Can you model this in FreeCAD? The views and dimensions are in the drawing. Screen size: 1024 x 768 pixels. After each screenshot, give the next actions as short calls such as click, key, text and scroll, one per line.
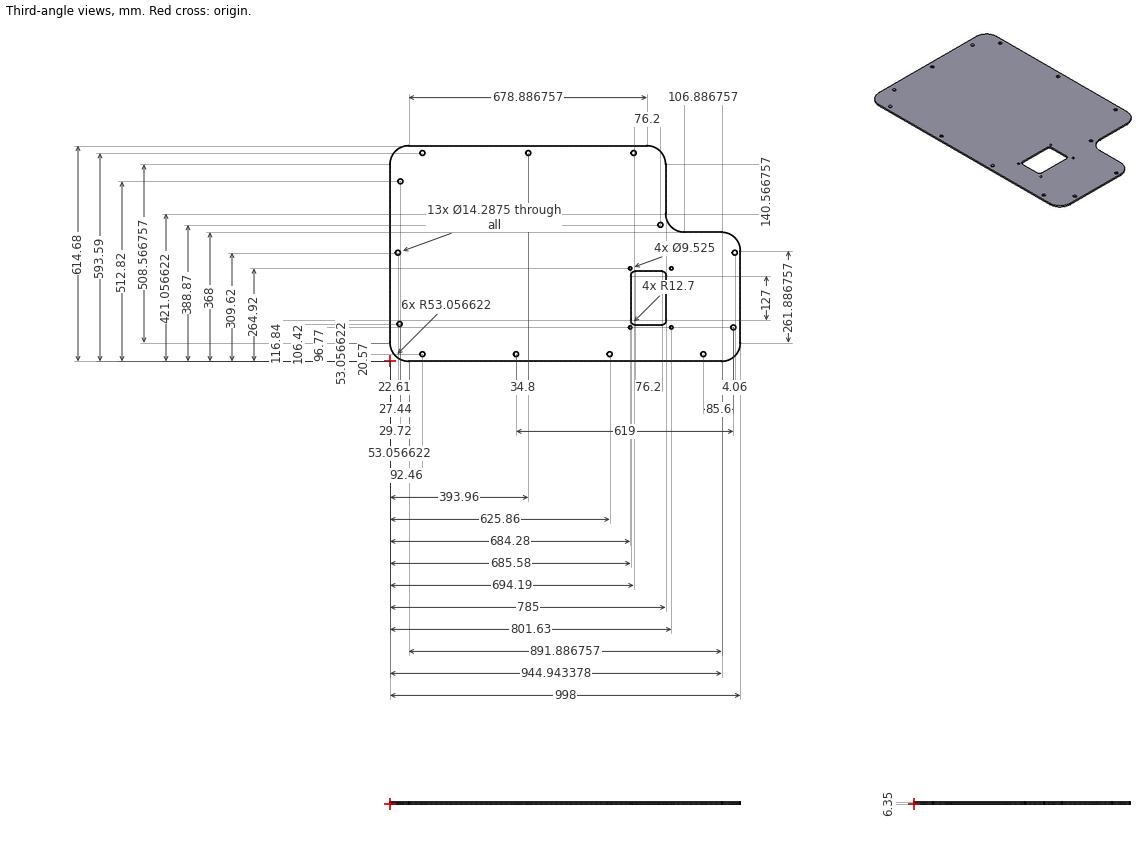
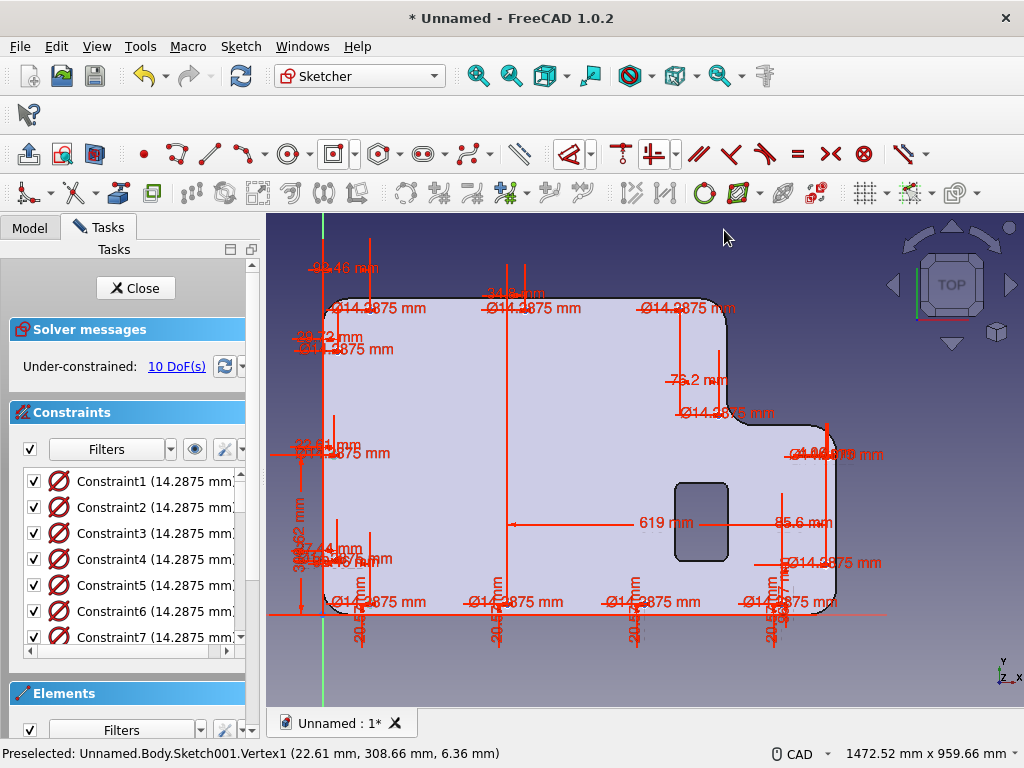
click(338, 351)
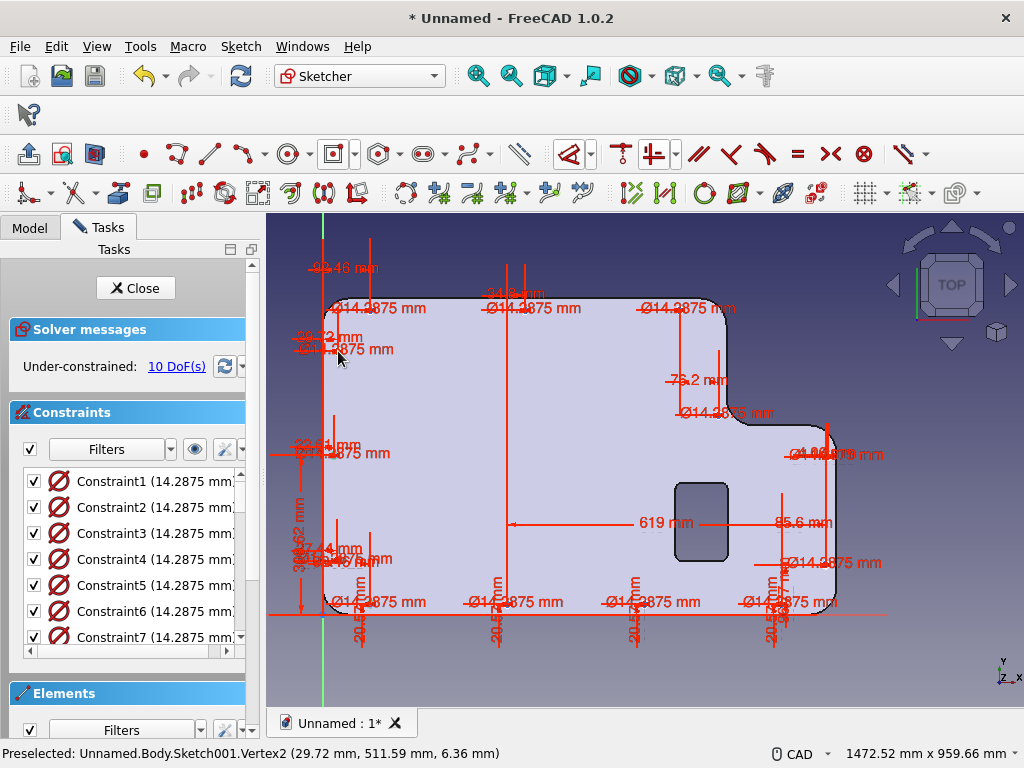
click(590, 154)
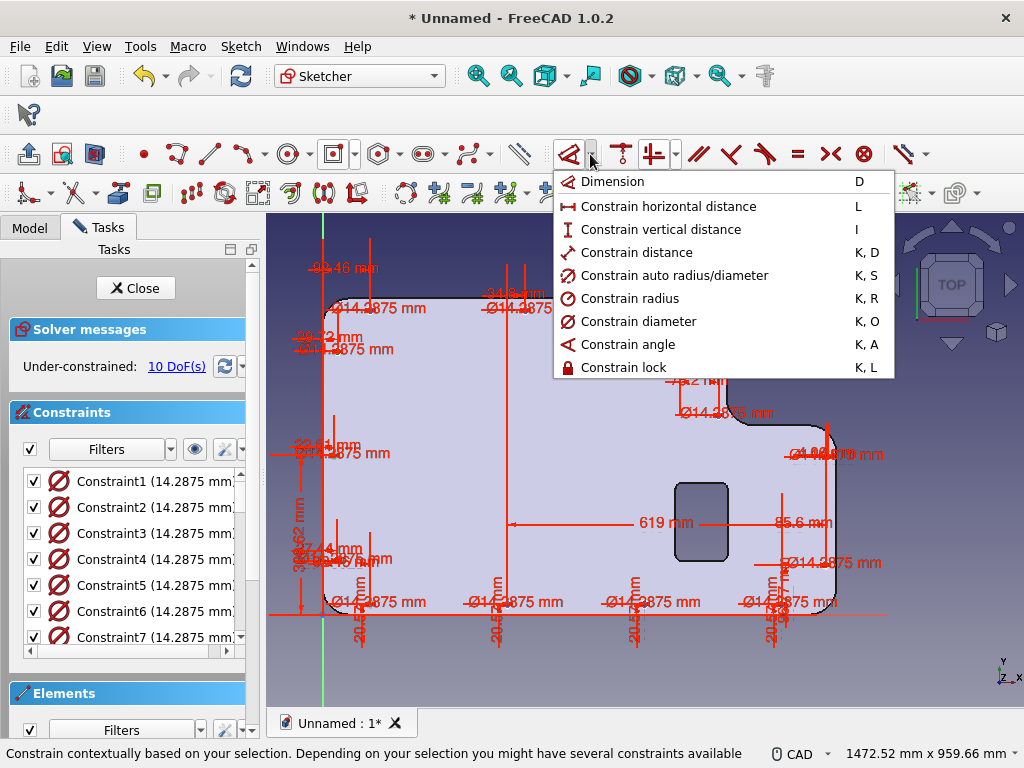
click(724, 230)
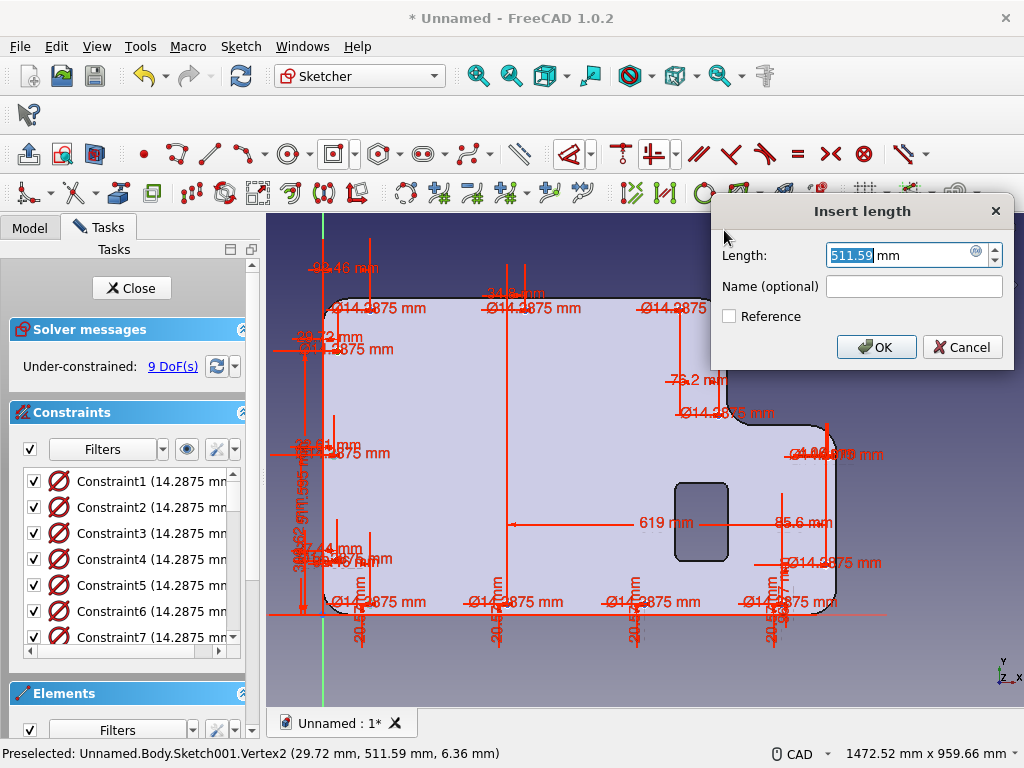
text(512.82)
key(Return)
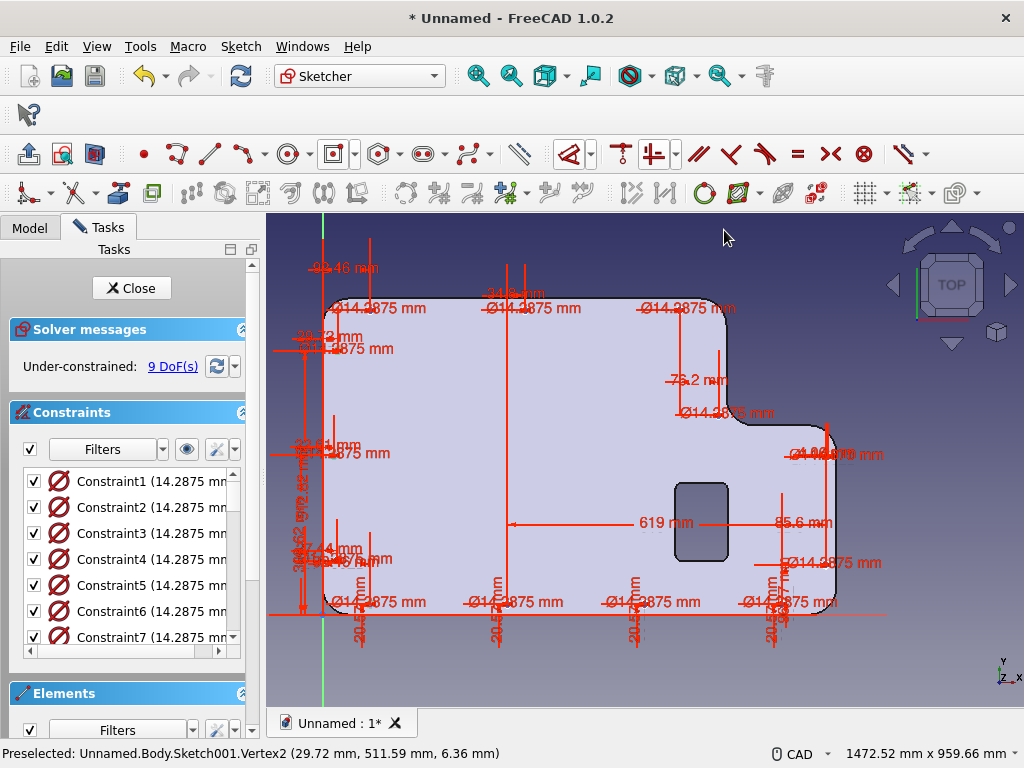
click(337, 561)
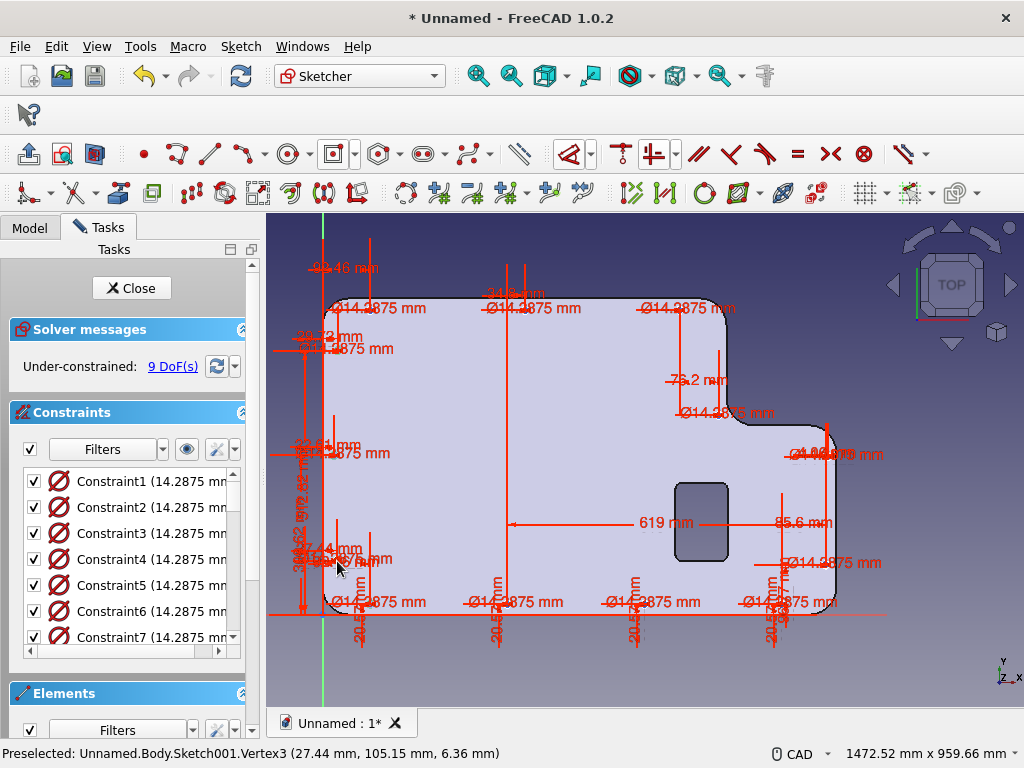
key(i)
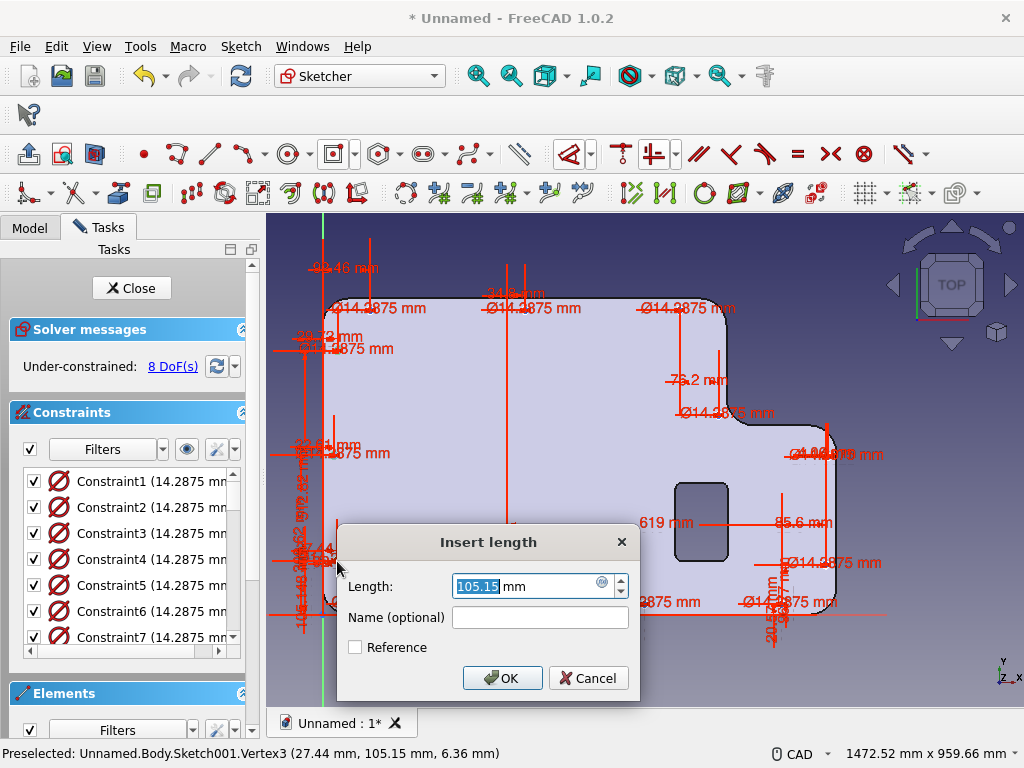
text(106.42)
key(Return)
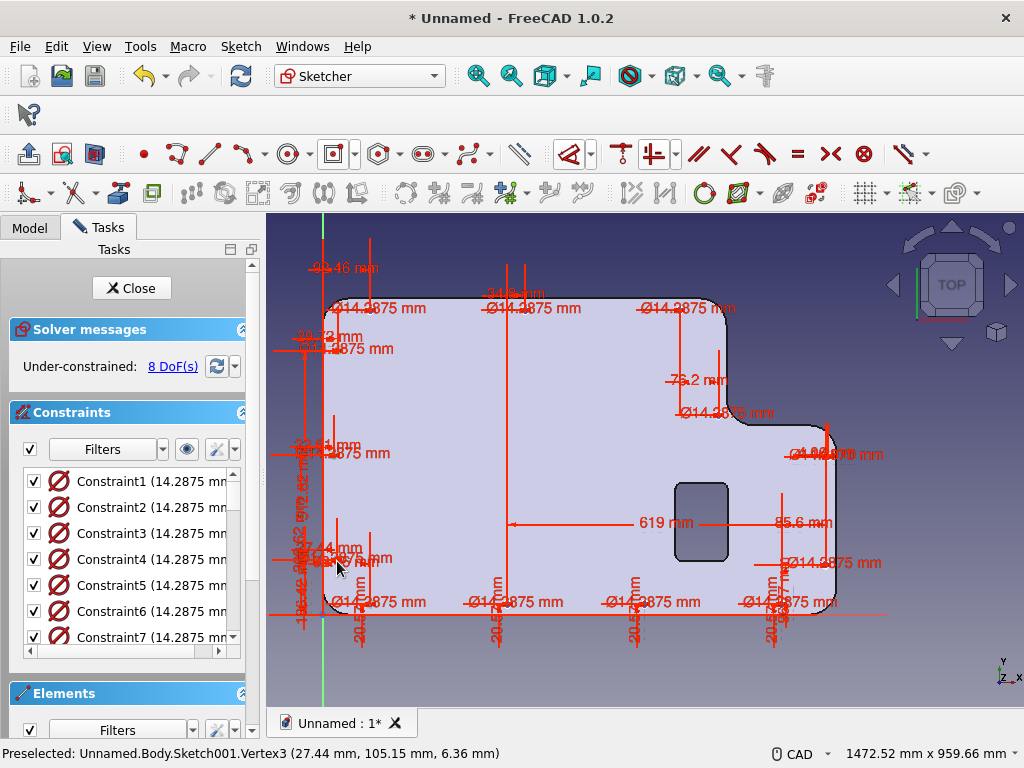
click(370, 310)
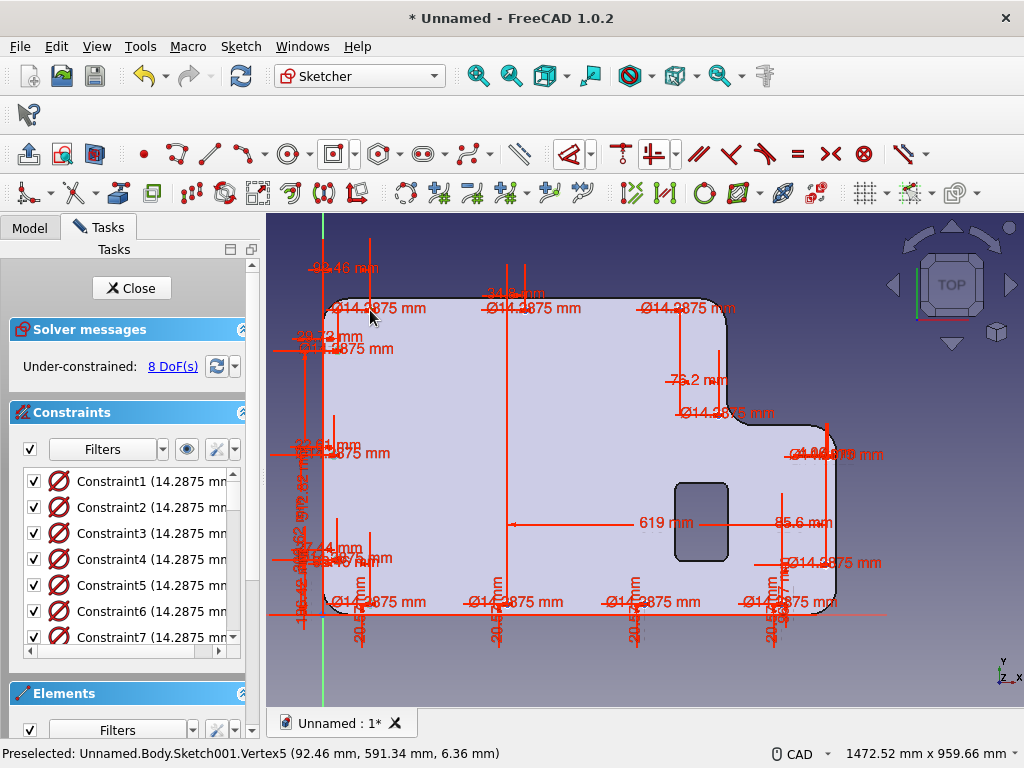
key(i)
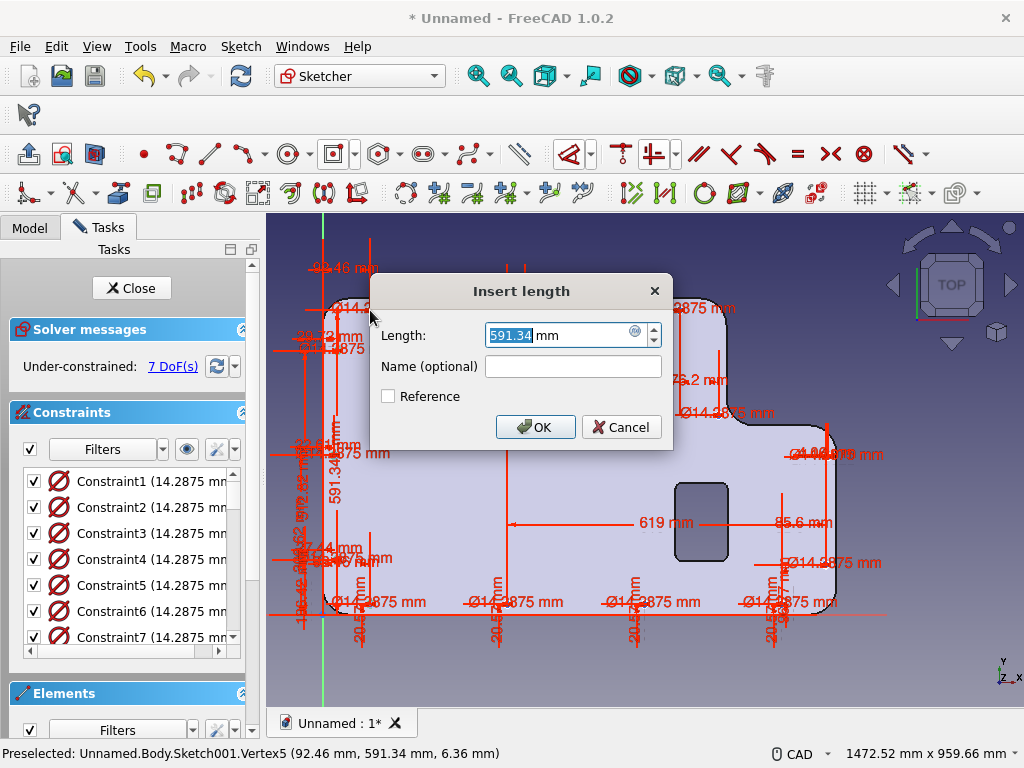
text(593.59)
key(Return)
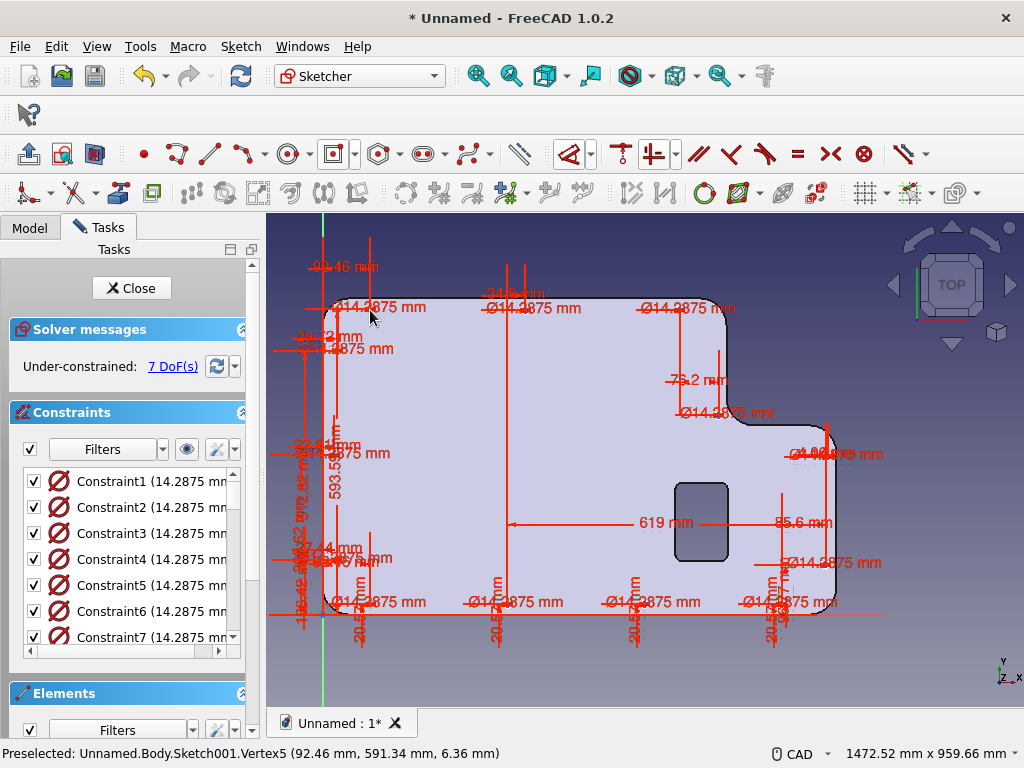
click(680, 310)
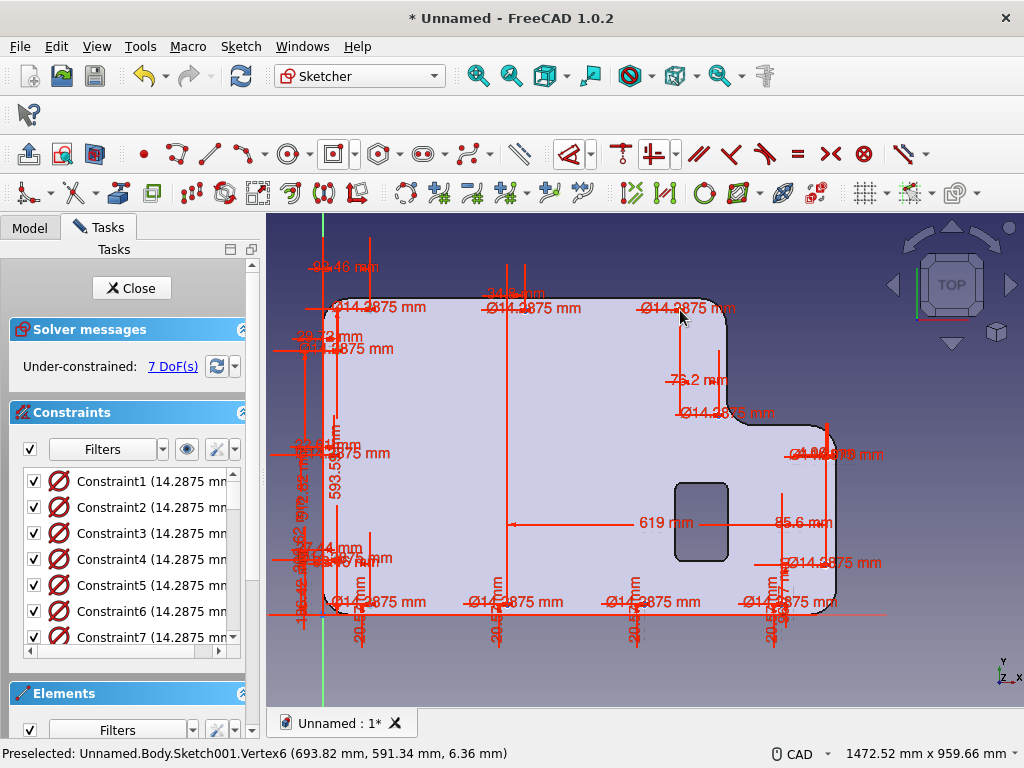
click(590, 154)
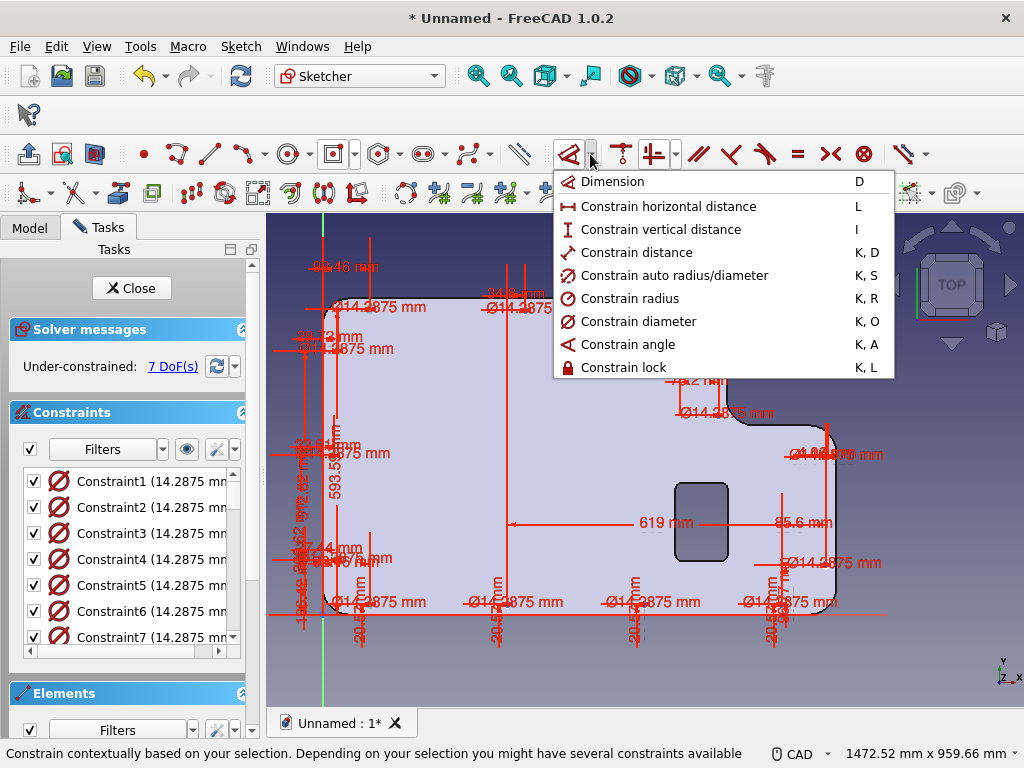
click(724, 206)